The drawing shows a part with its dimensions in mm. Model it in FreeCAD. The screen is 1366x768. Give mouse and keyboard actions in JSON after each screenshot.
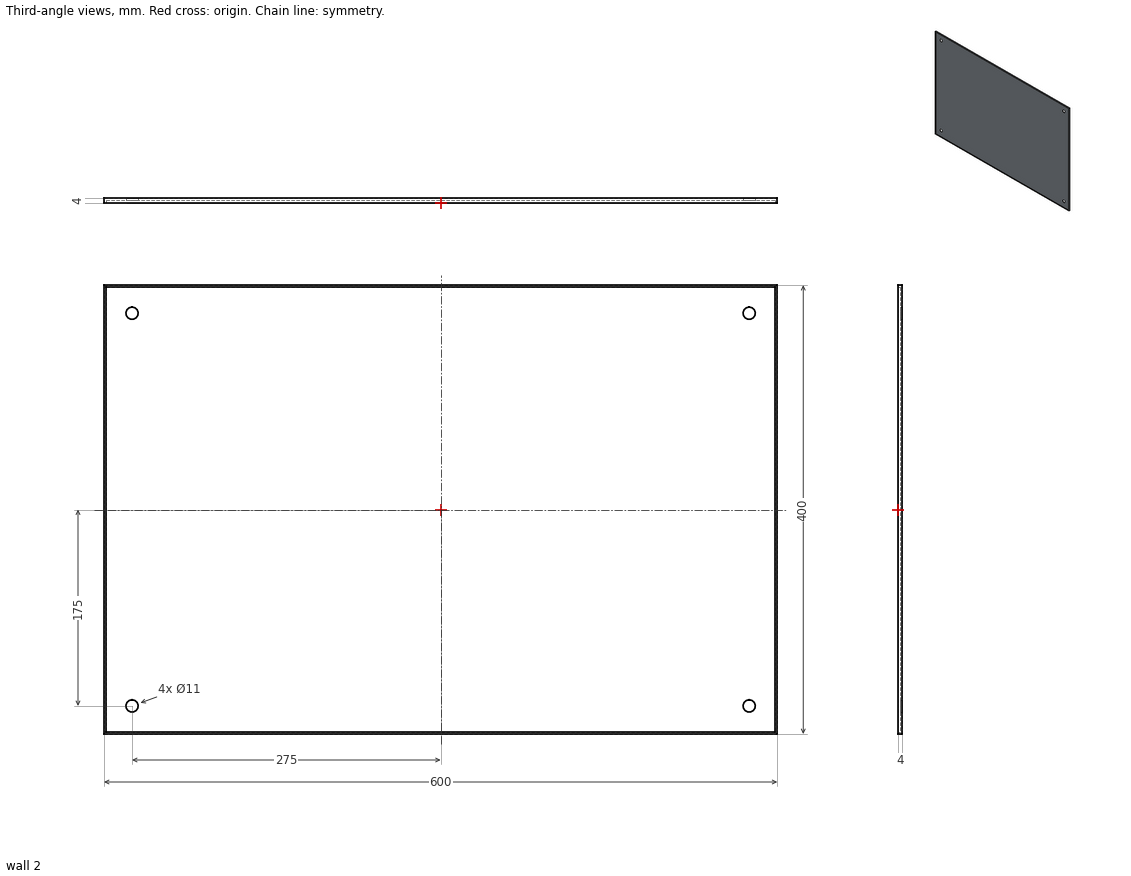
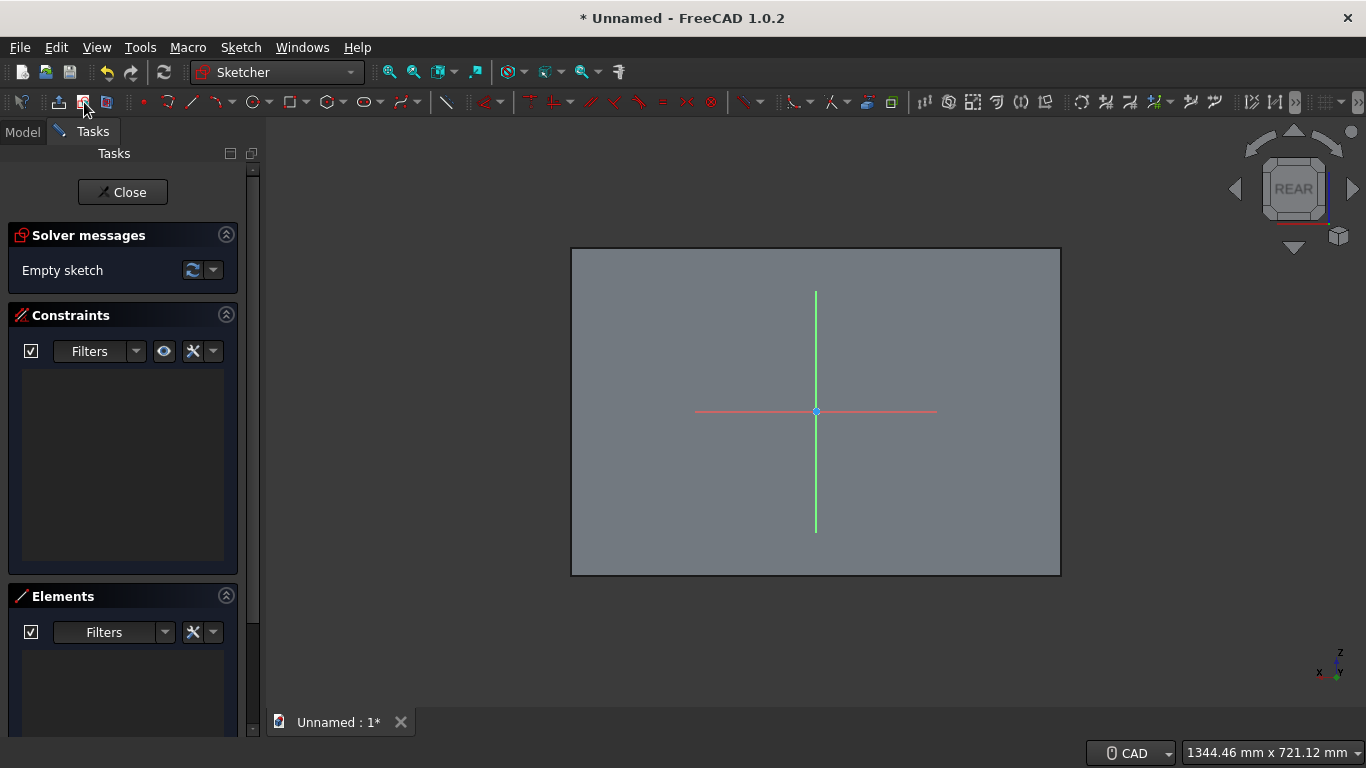
{"action": "key", "text": "g c"}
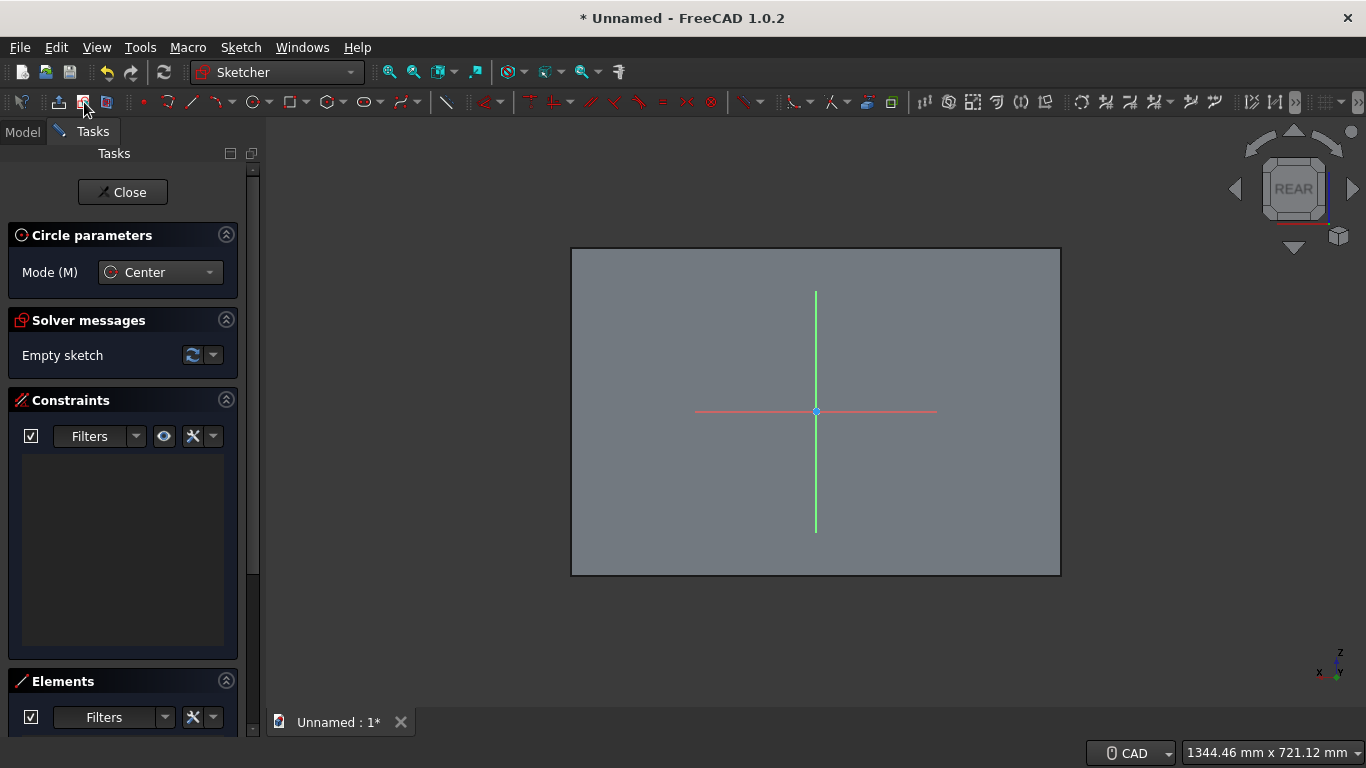
{"action": "scroll", "coordinate": [1041, 555], "scroll_direction": "up", "scroll_amount": 9}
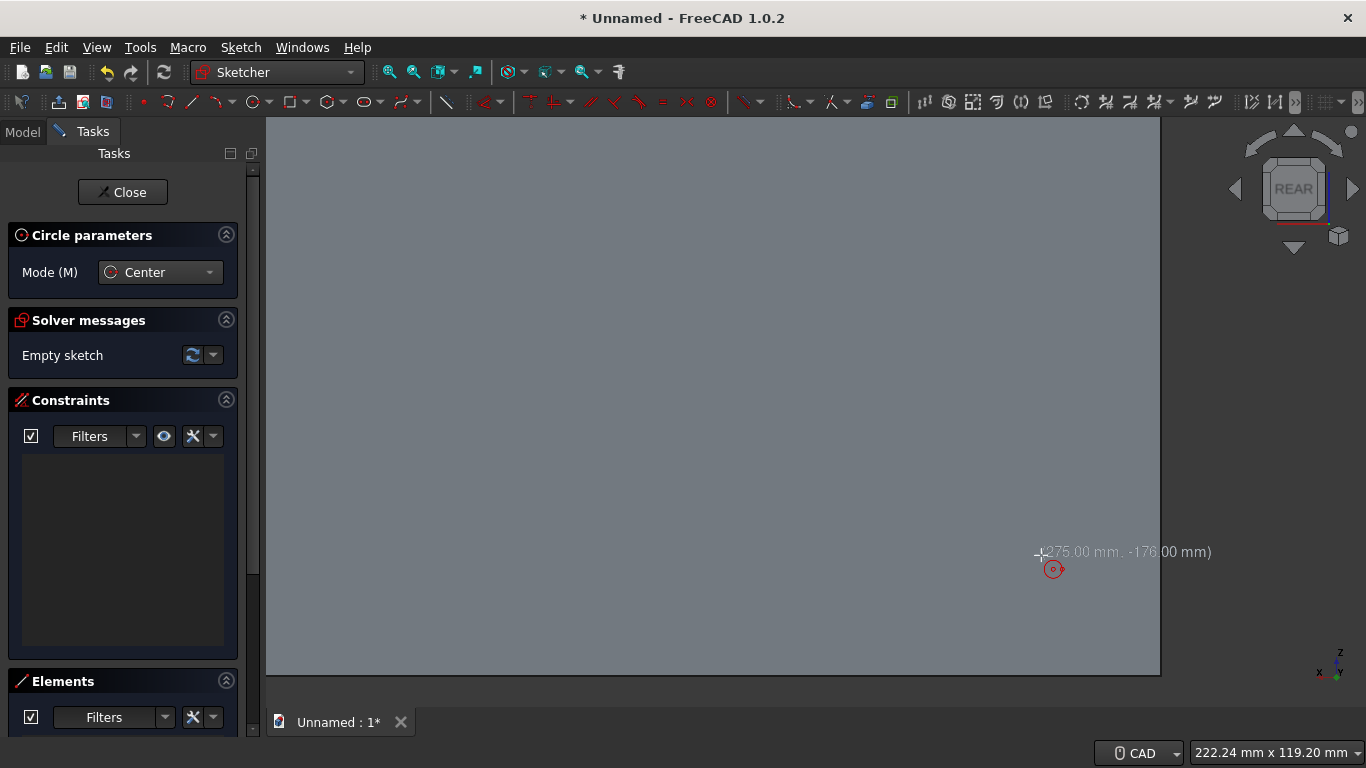
{"action": "scroll", "coordinate": [1018, 596], "scroll_direction": "down", "scroll_amount": 8}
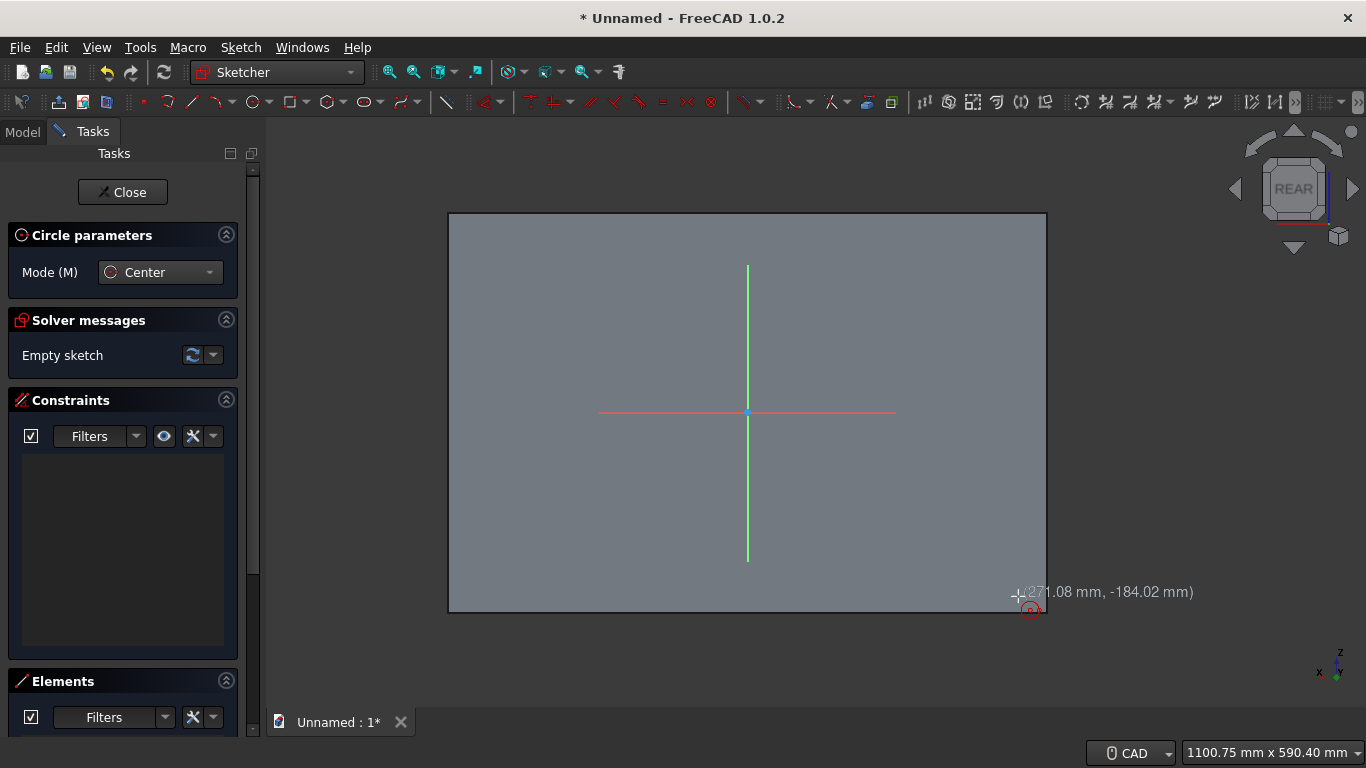
{"action": "left_click", "coordinate": [1022, 588]}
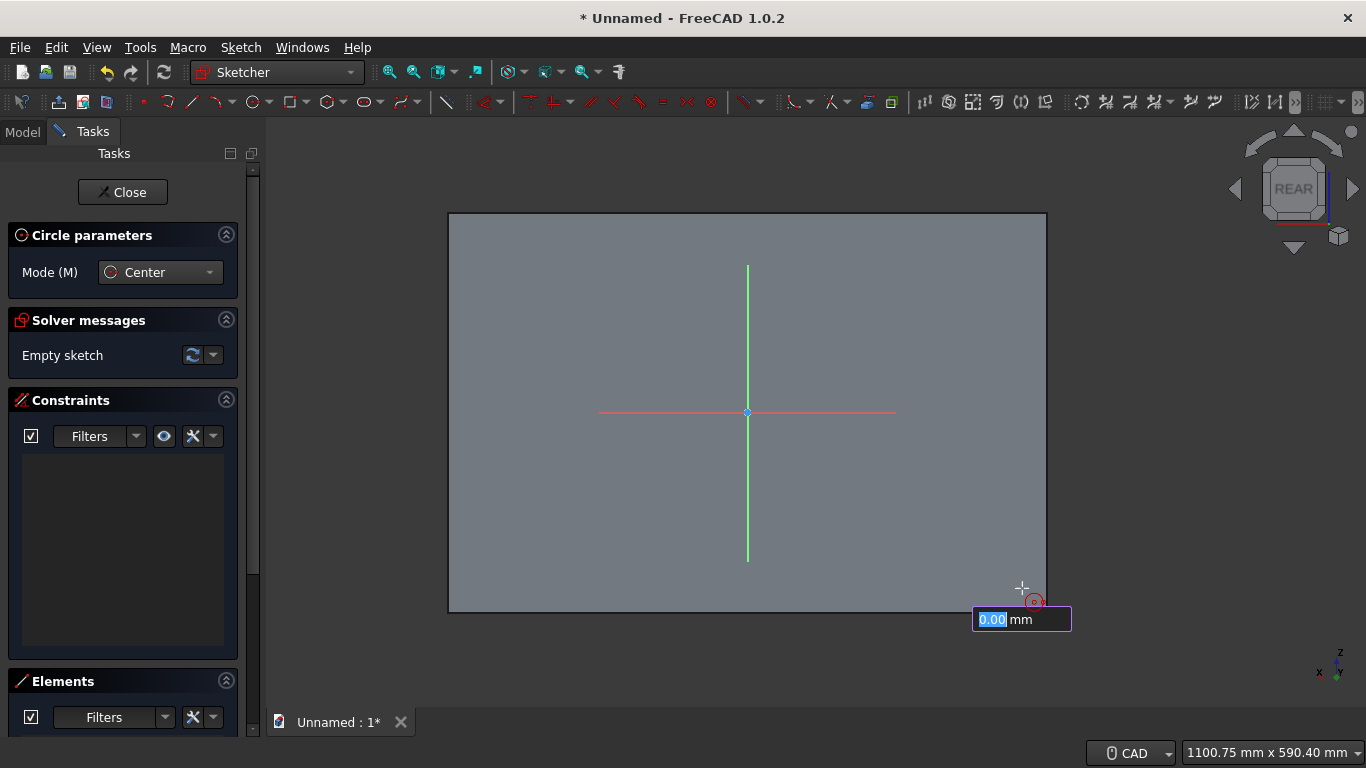
{"action": "scroll", "coordinate": [1026, 584], "scroll_direction": "up", "scroll_amount": 6}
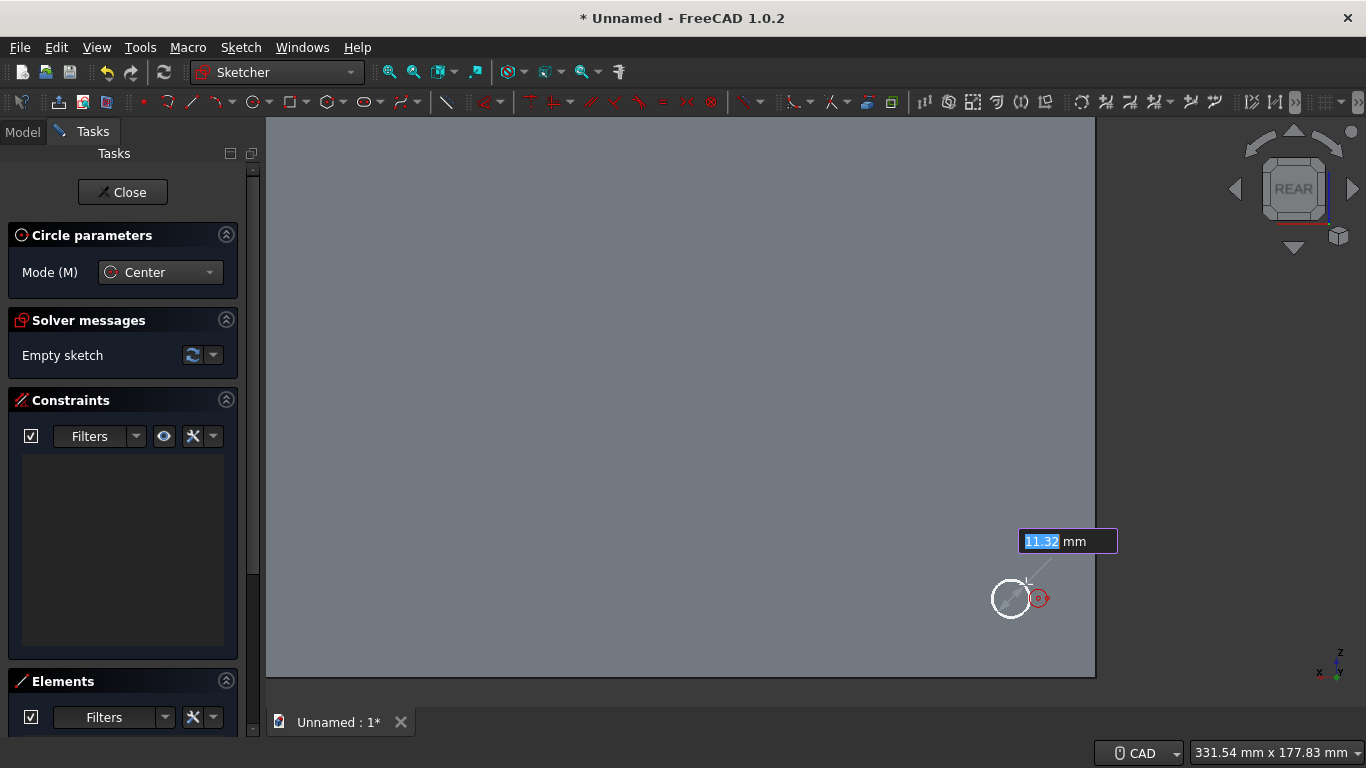
{"action": "left_click", "coordinate": [1026, 582]}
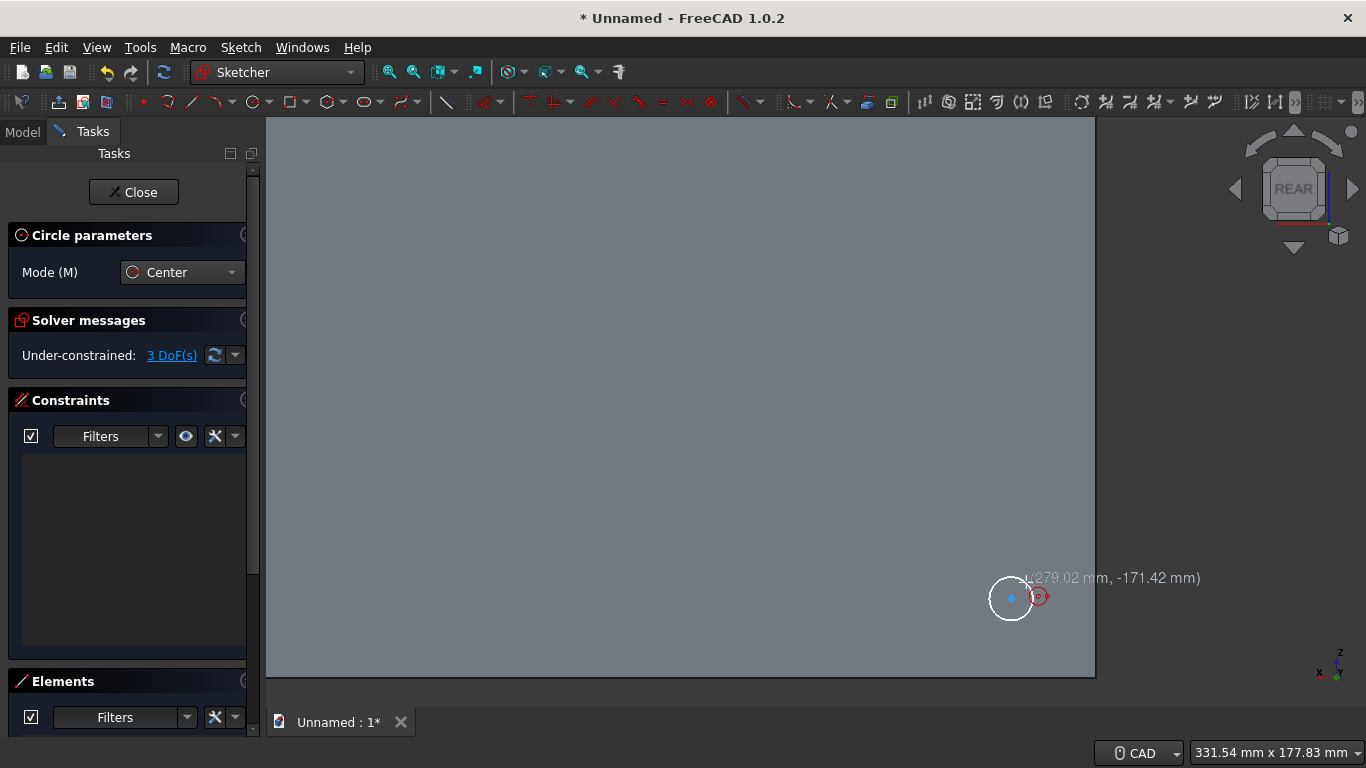
{"action": "scroll", "coordinate": [1026, 583], "scroll_direction": "down", "scroll_amount": 6}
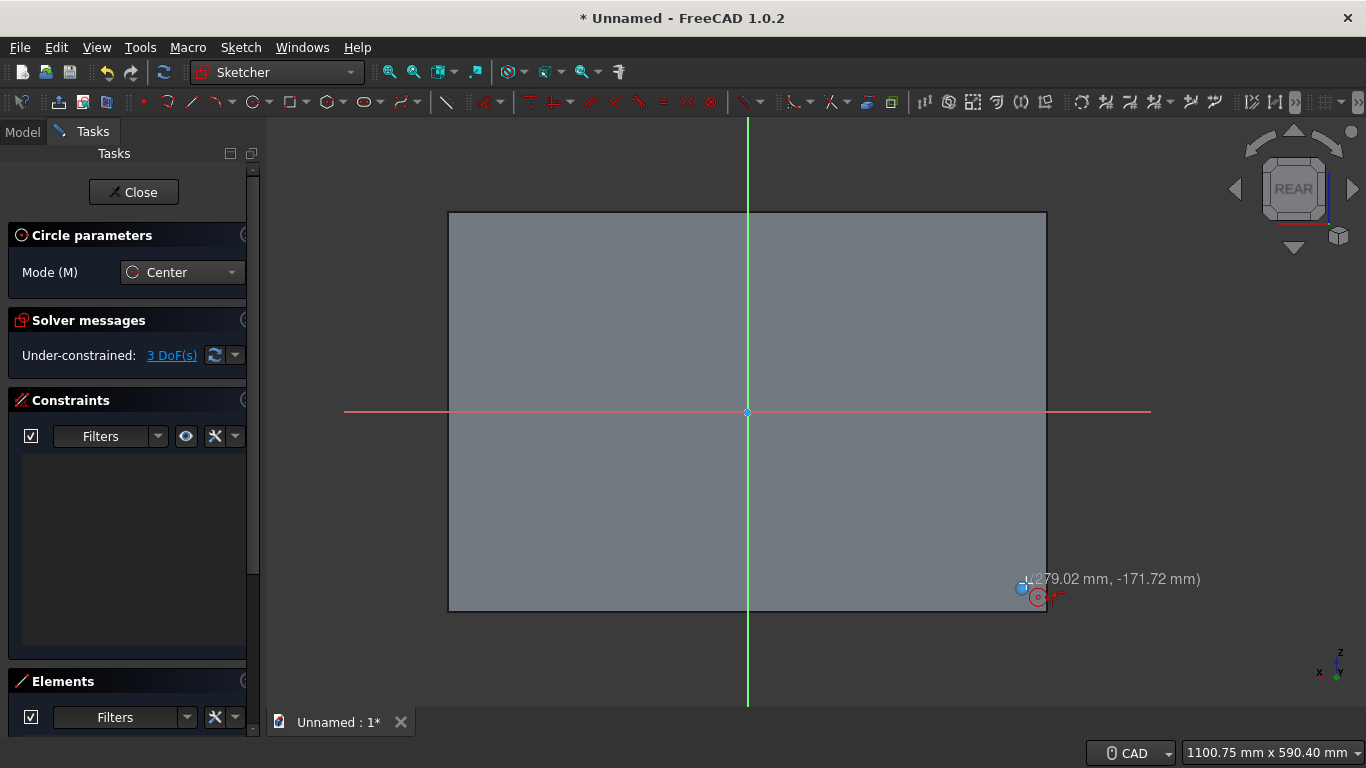
{"action": "scroll", "coordinate": [473, 587], "scroll_direction": "up", "scroll_amount": 8}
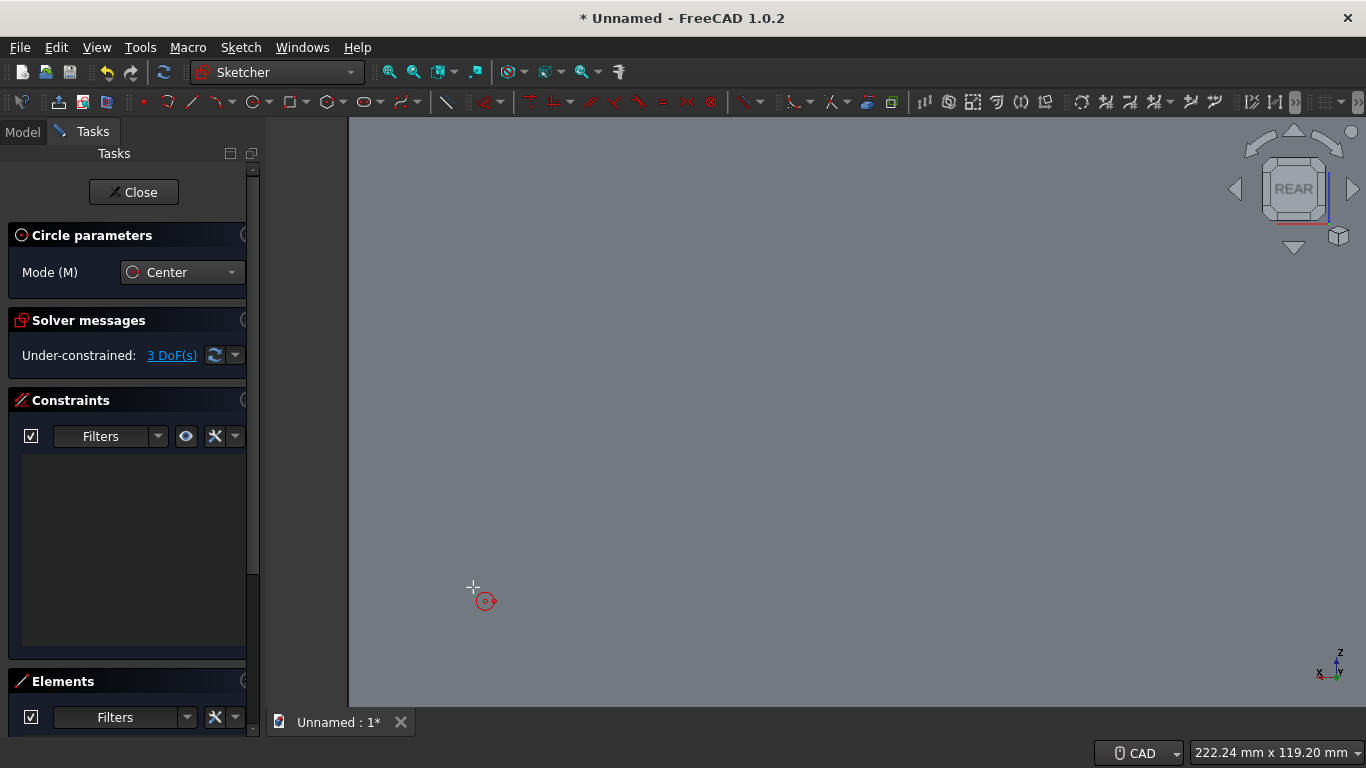
{"action": "scroll", "coordinate": [473, 587], "scroll_direction": "down", "scroll_amount": 8}